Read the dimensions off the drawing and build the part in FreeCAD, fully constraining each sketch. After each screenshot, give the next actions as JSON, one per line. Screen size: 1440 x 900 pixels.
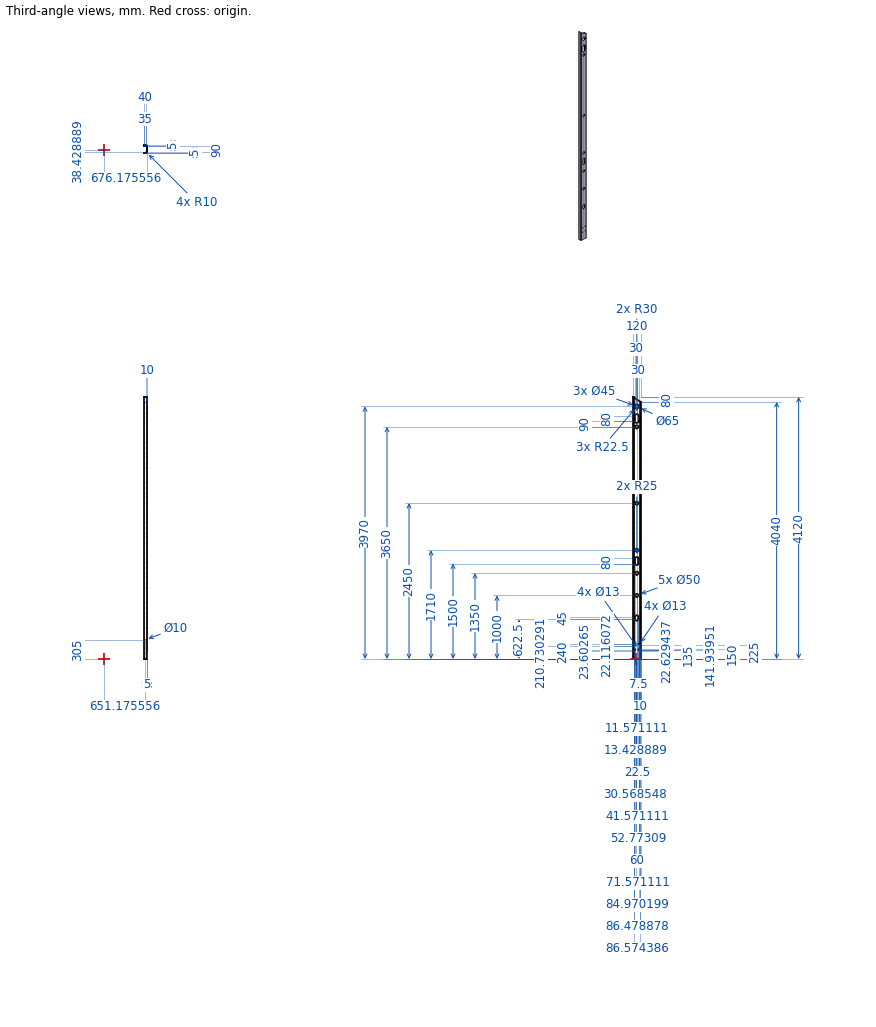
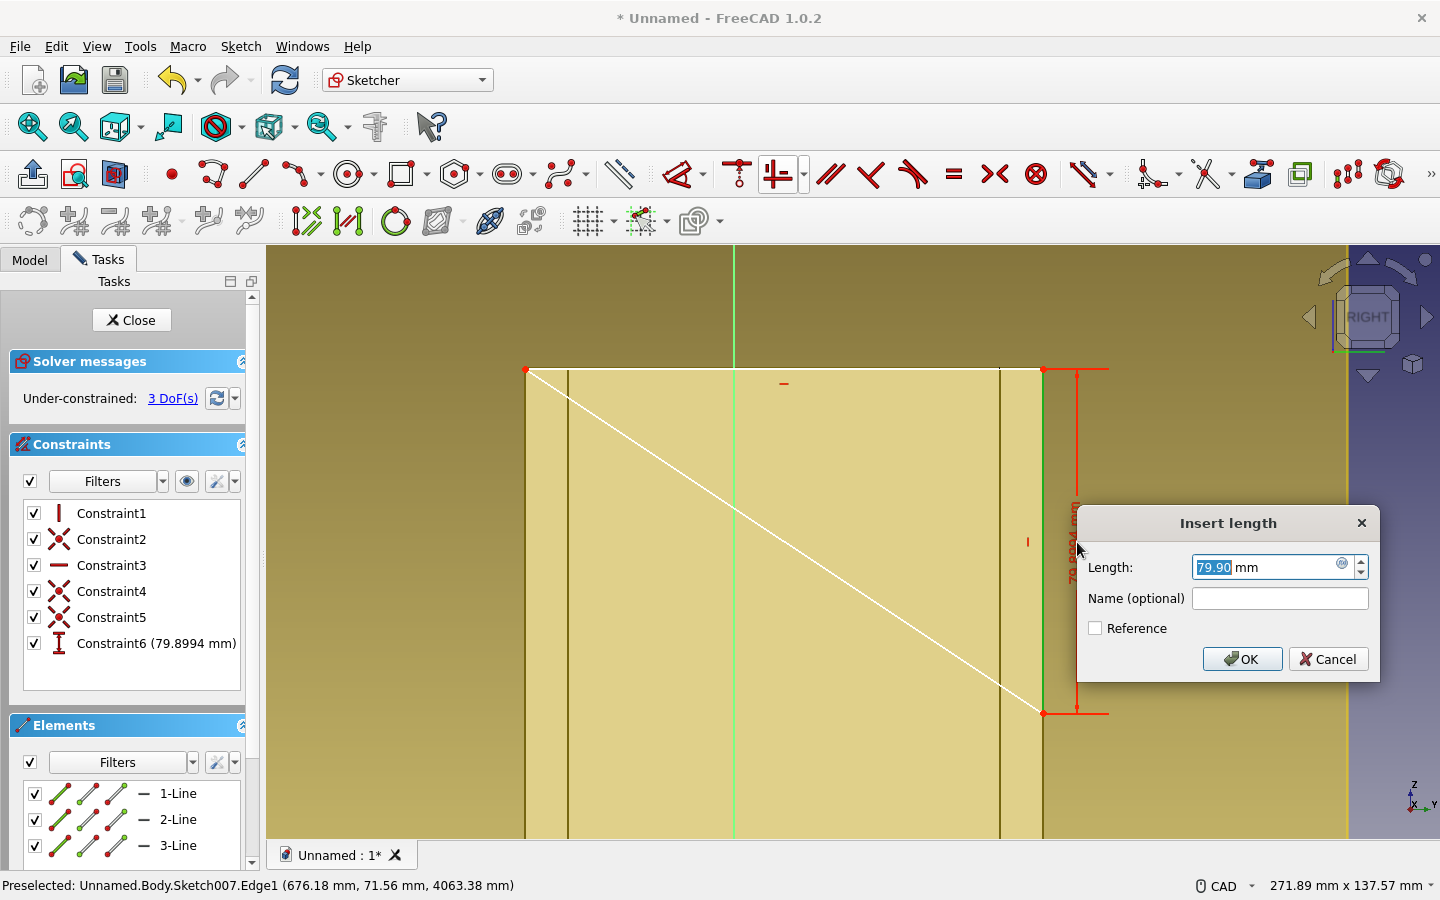
{"action": "type", "text": "80"}
{"action": "key", "text": "Return"}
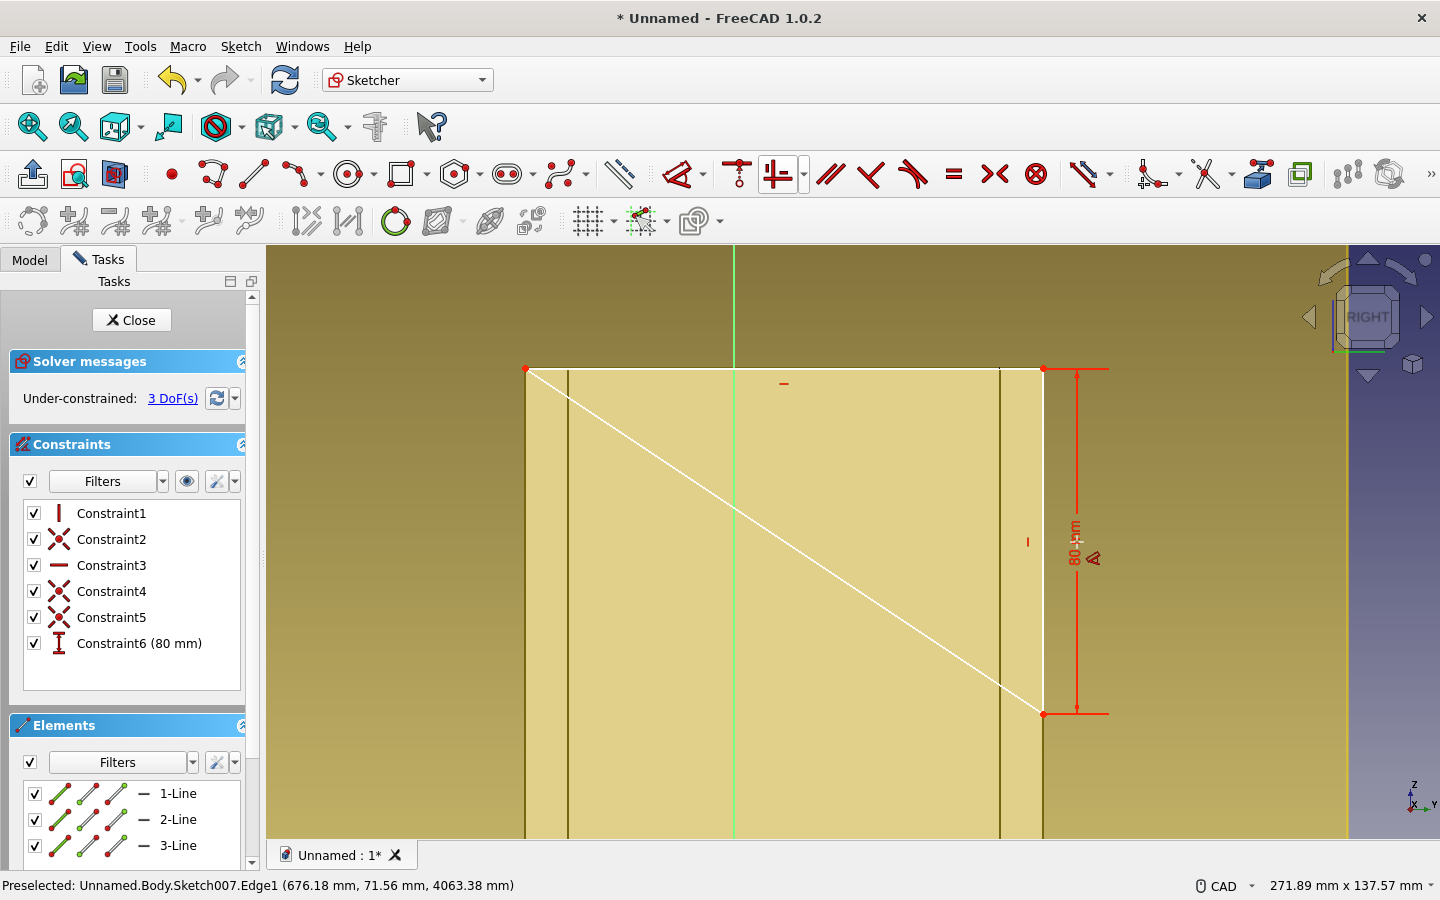
{"action": "left_click", "coordinate": [888, 369]}
{"action": "left_click", "coordinate": [784, 335]}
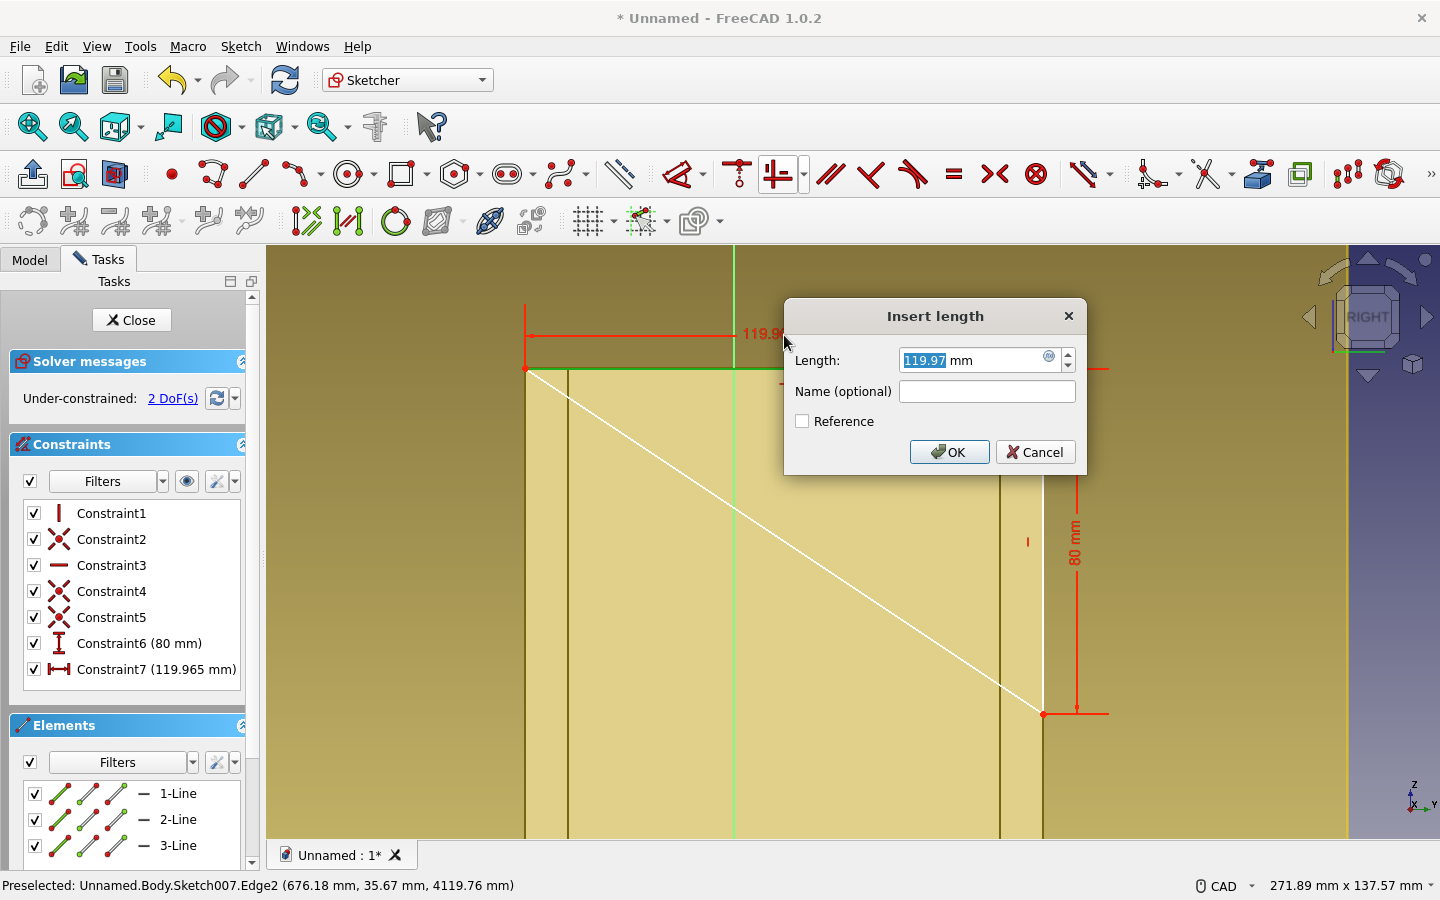
{"action": "type", "text": "120"}
{"action": "key", "text": "Return"}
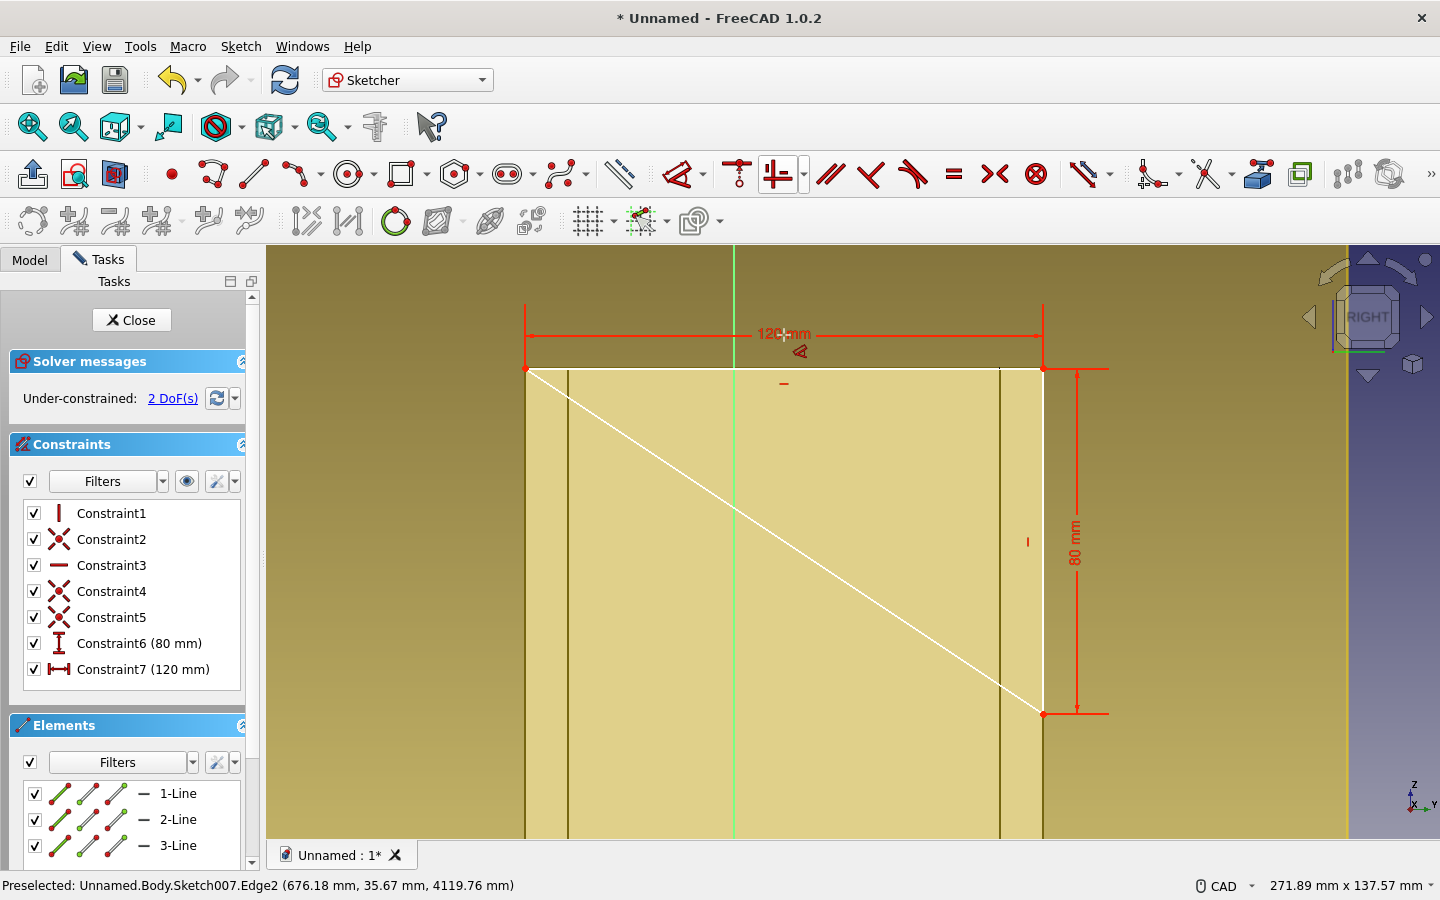
{"action": "left_click", "coordinate": [1043, 714]}
{"action": "left_click", "coordinate": [1077, 763]}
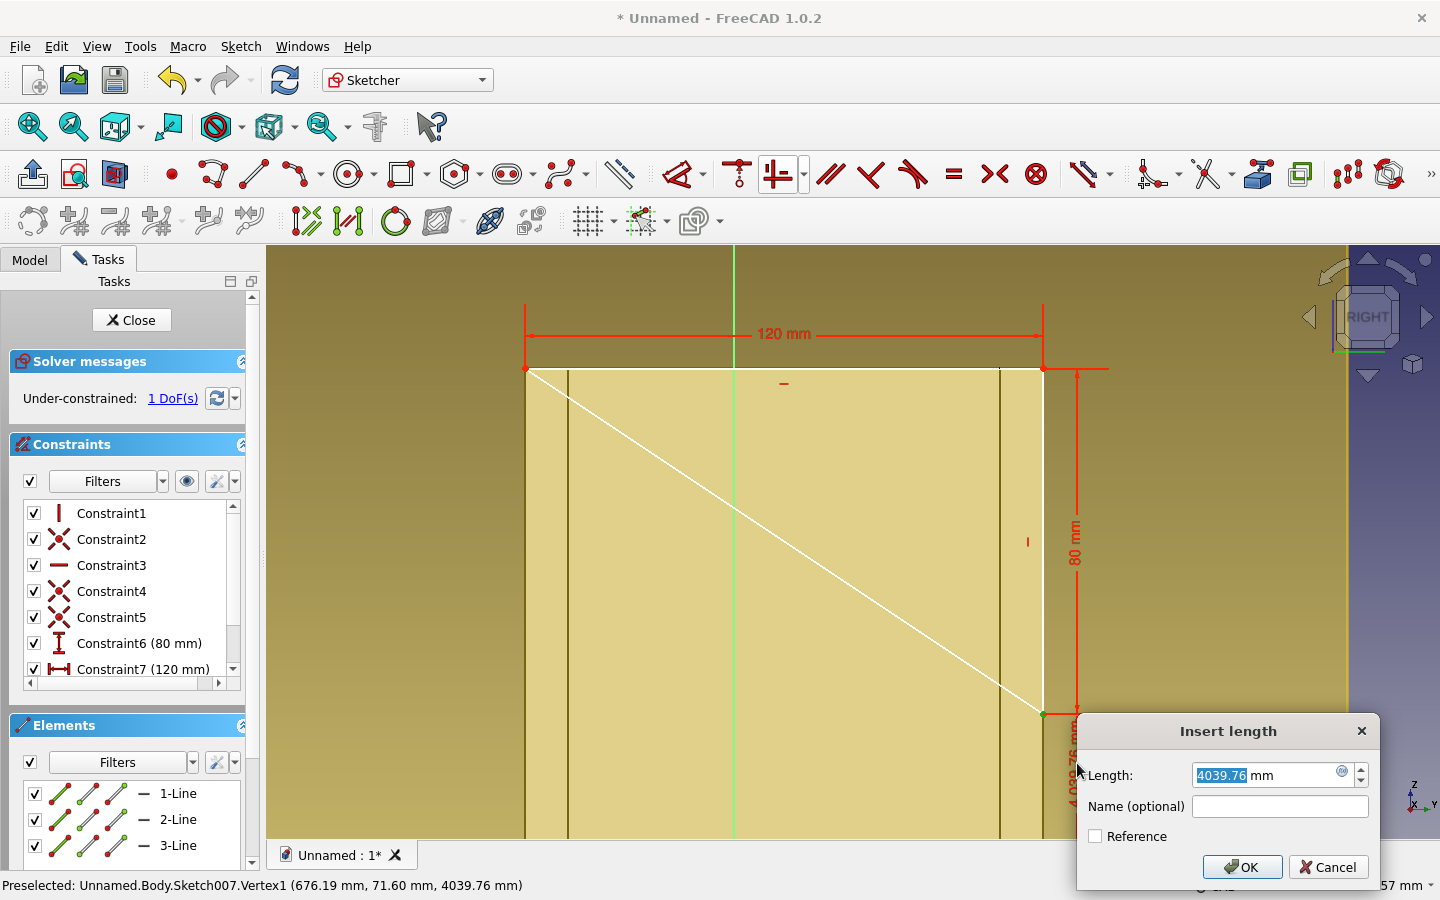
{"action": "type", "text": "4040"}
{"action": "key", "text": "Return"}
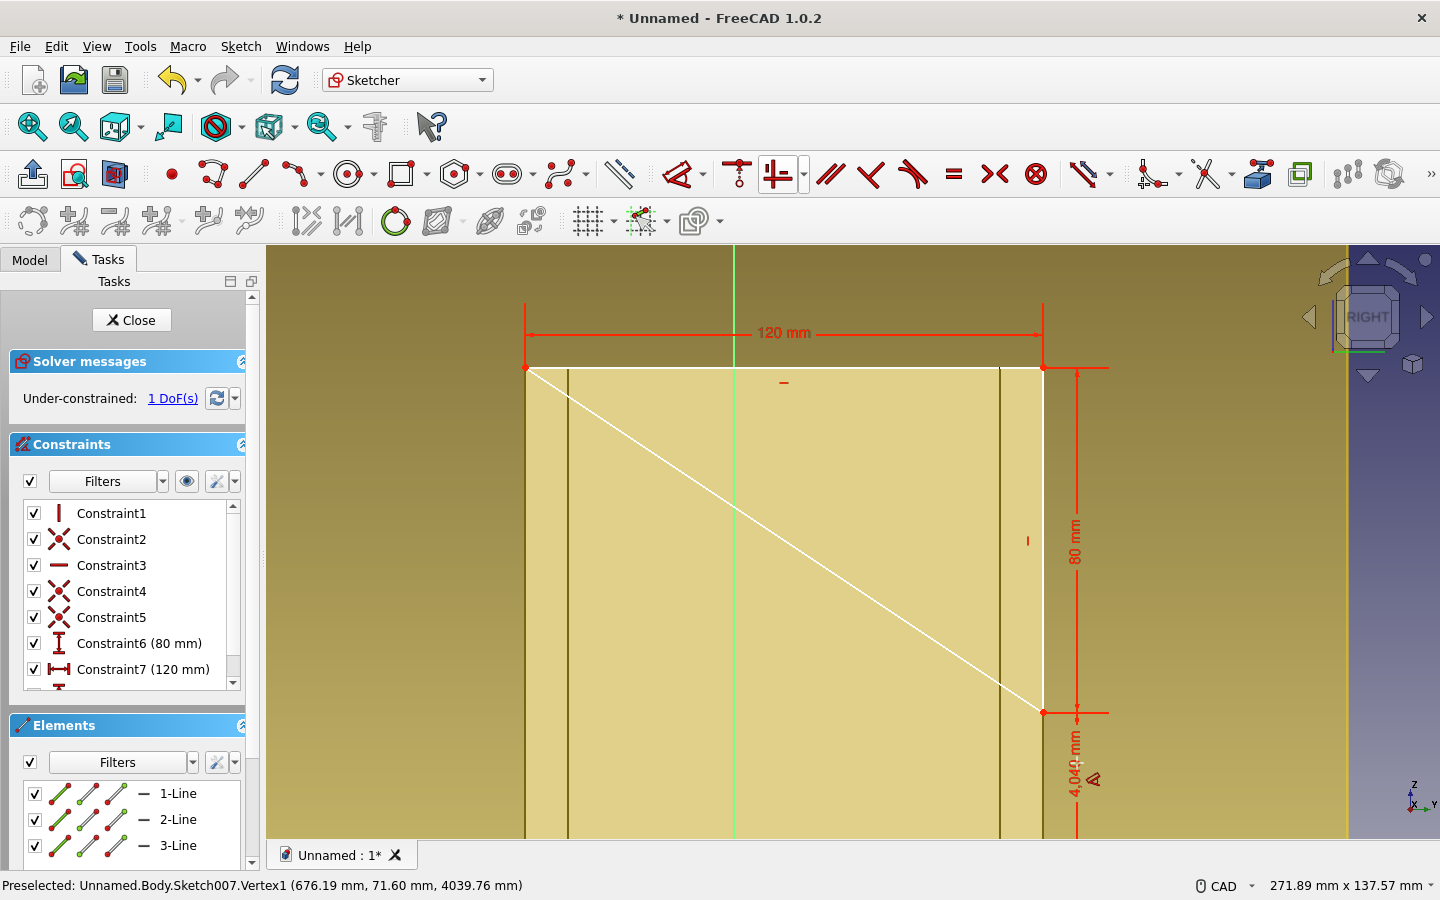
{"action": "left_click", "coordinate": [1043, 713]}
{"action": "left_click", "coordinate": [889, 679]}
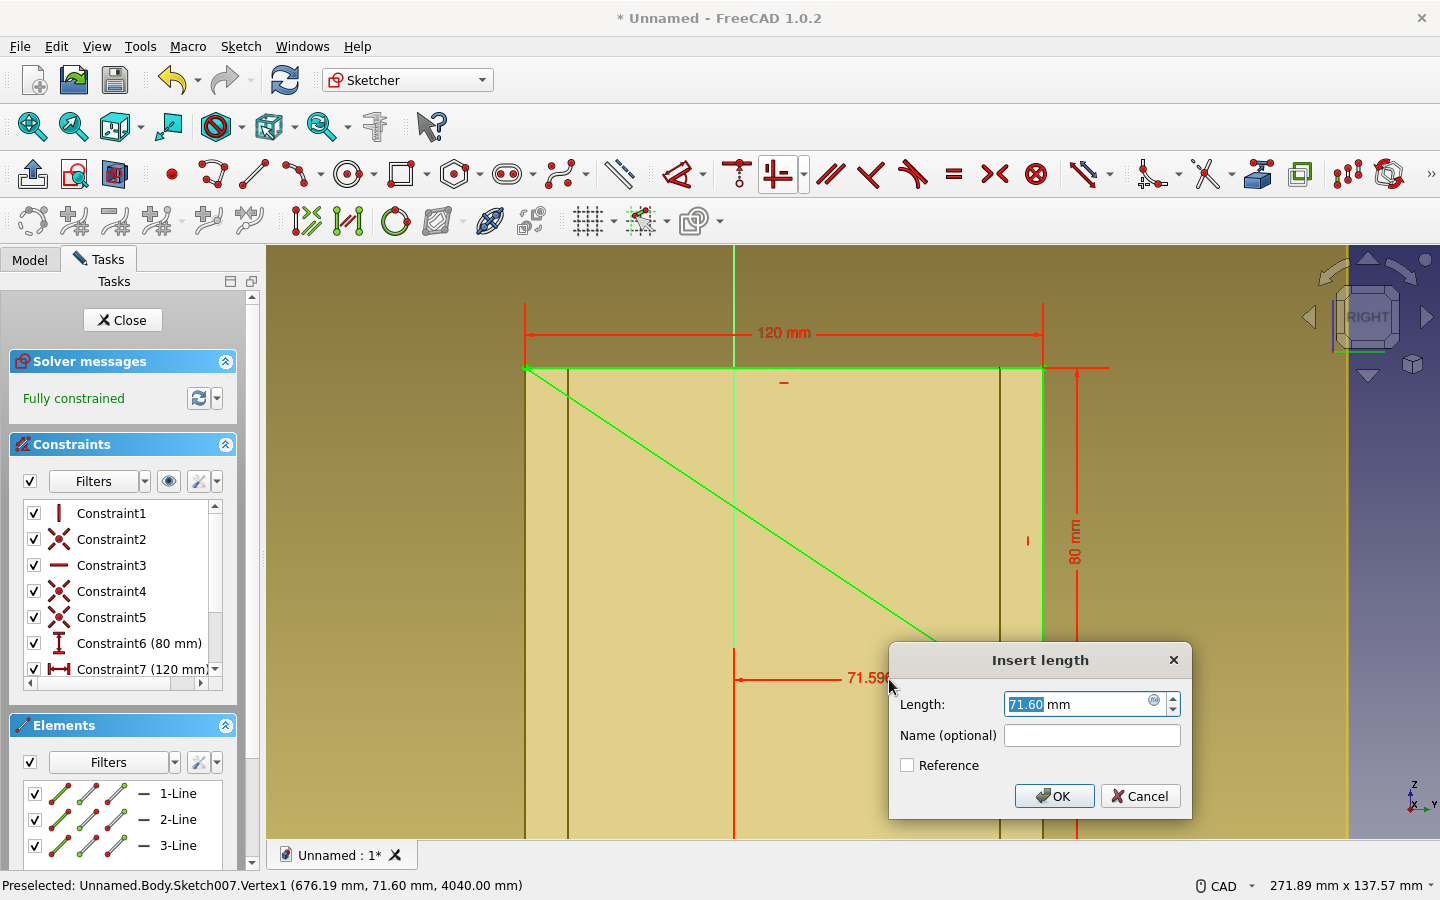
{"action": "type", "text": "71.571111"}
{"action": "key", "text": "Return"}
{"action": "key", "text": "Escape"}